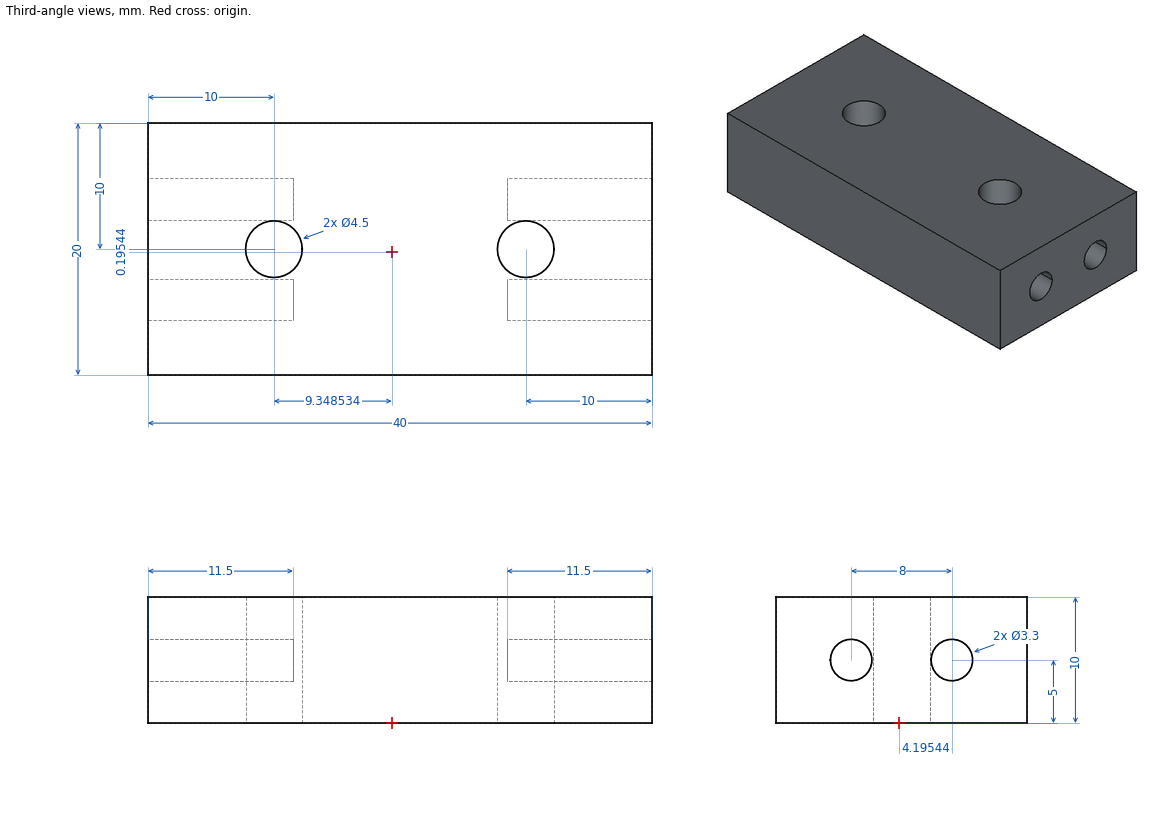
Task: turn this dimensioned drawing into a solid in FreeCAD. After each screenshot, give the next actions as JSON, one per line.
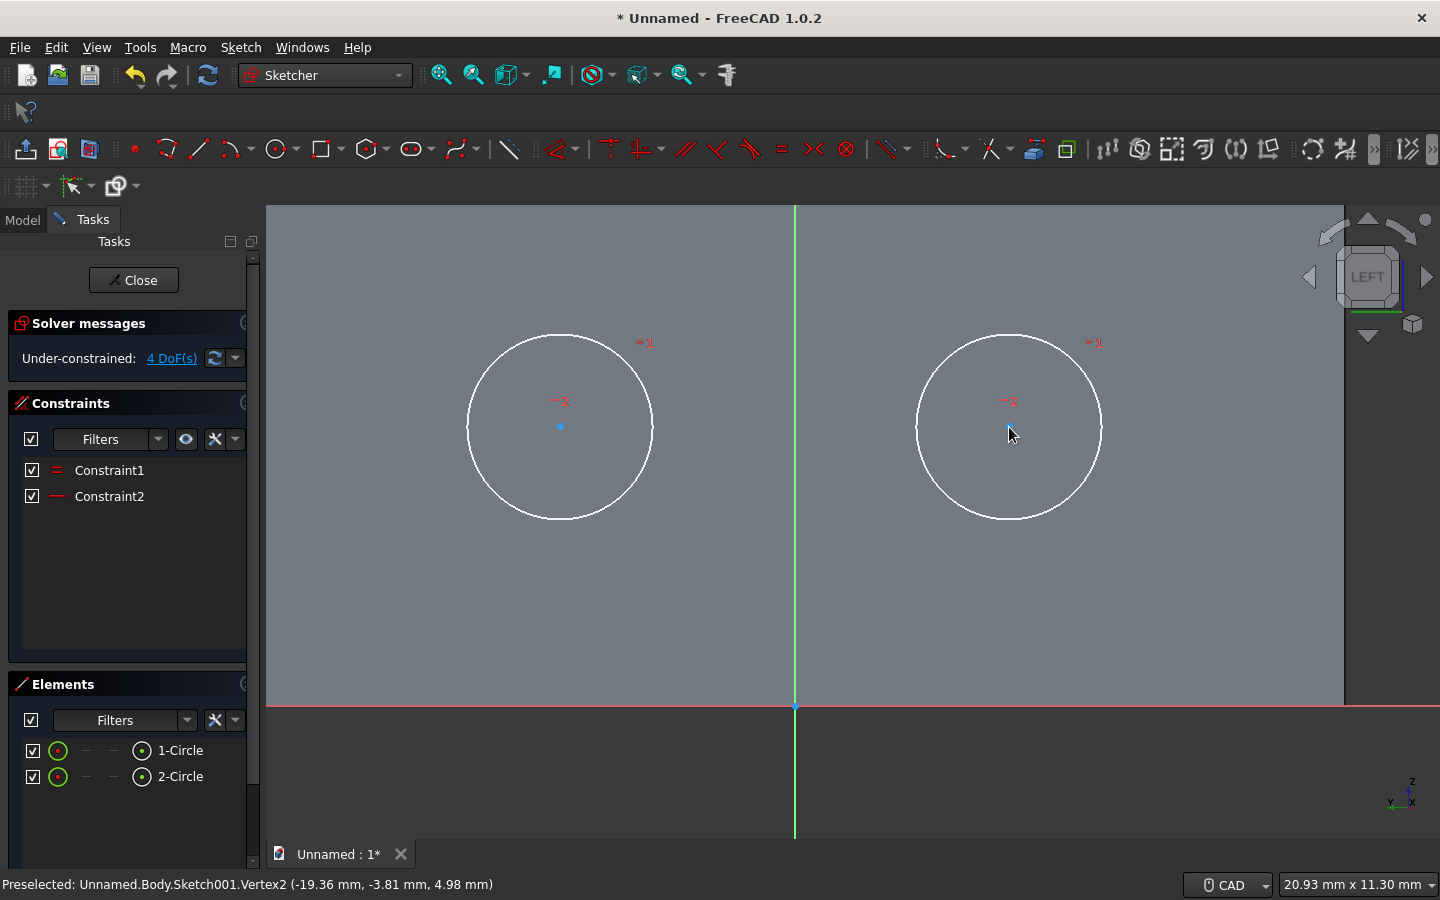
{"action": "left_click", "coordinate": [556, 150]}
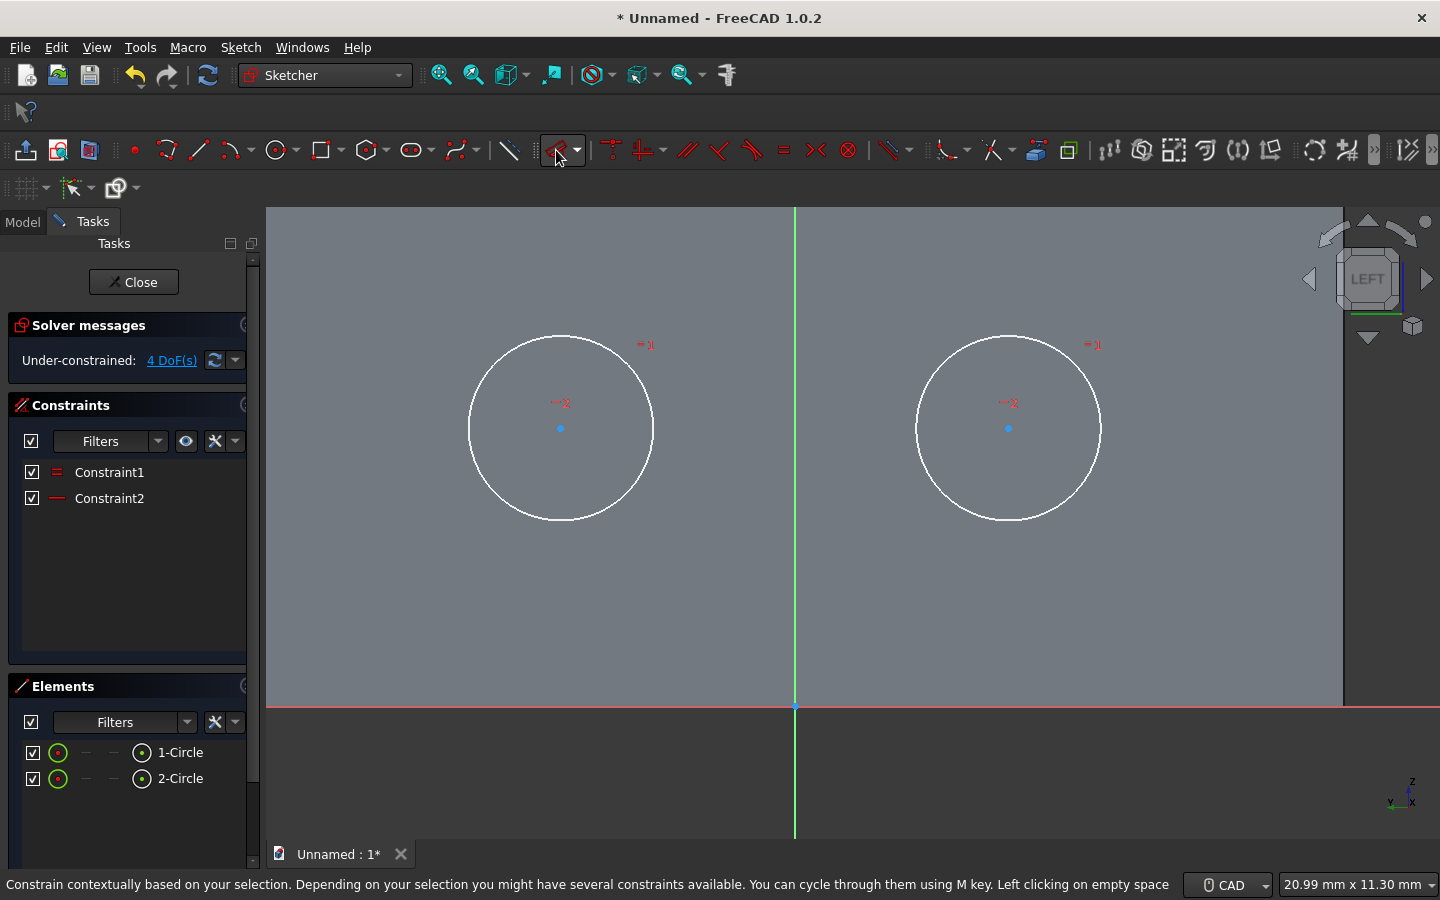
{"action": "left_click", "coordinate": [626, 363]}
{"action": "left_click", "coordinate": [649, 340]}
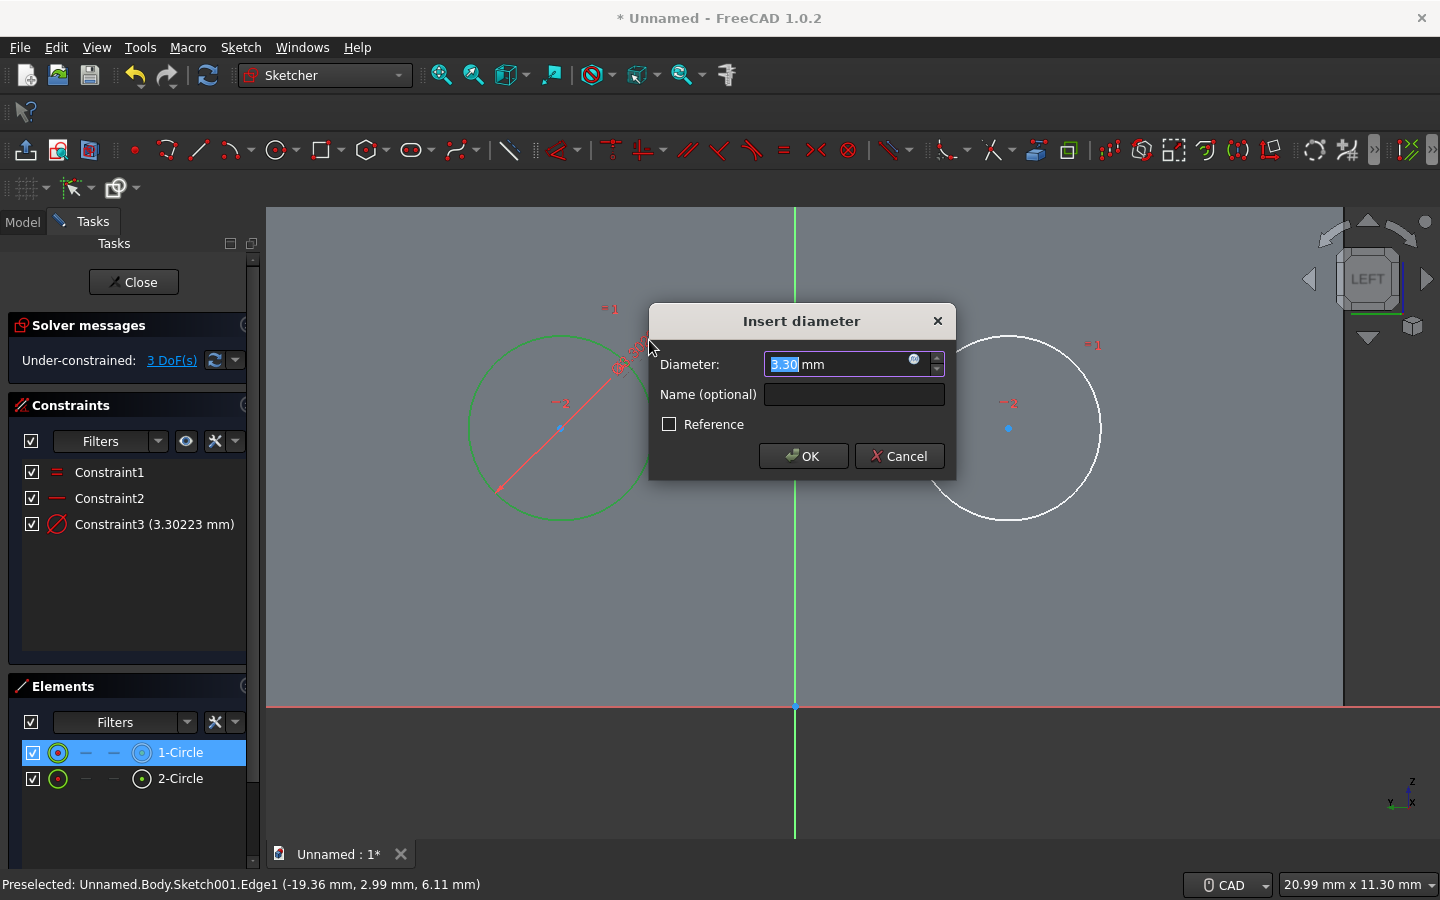
{"action": "type", "text": "3.3"}
{"action": "key", "text": "Return"}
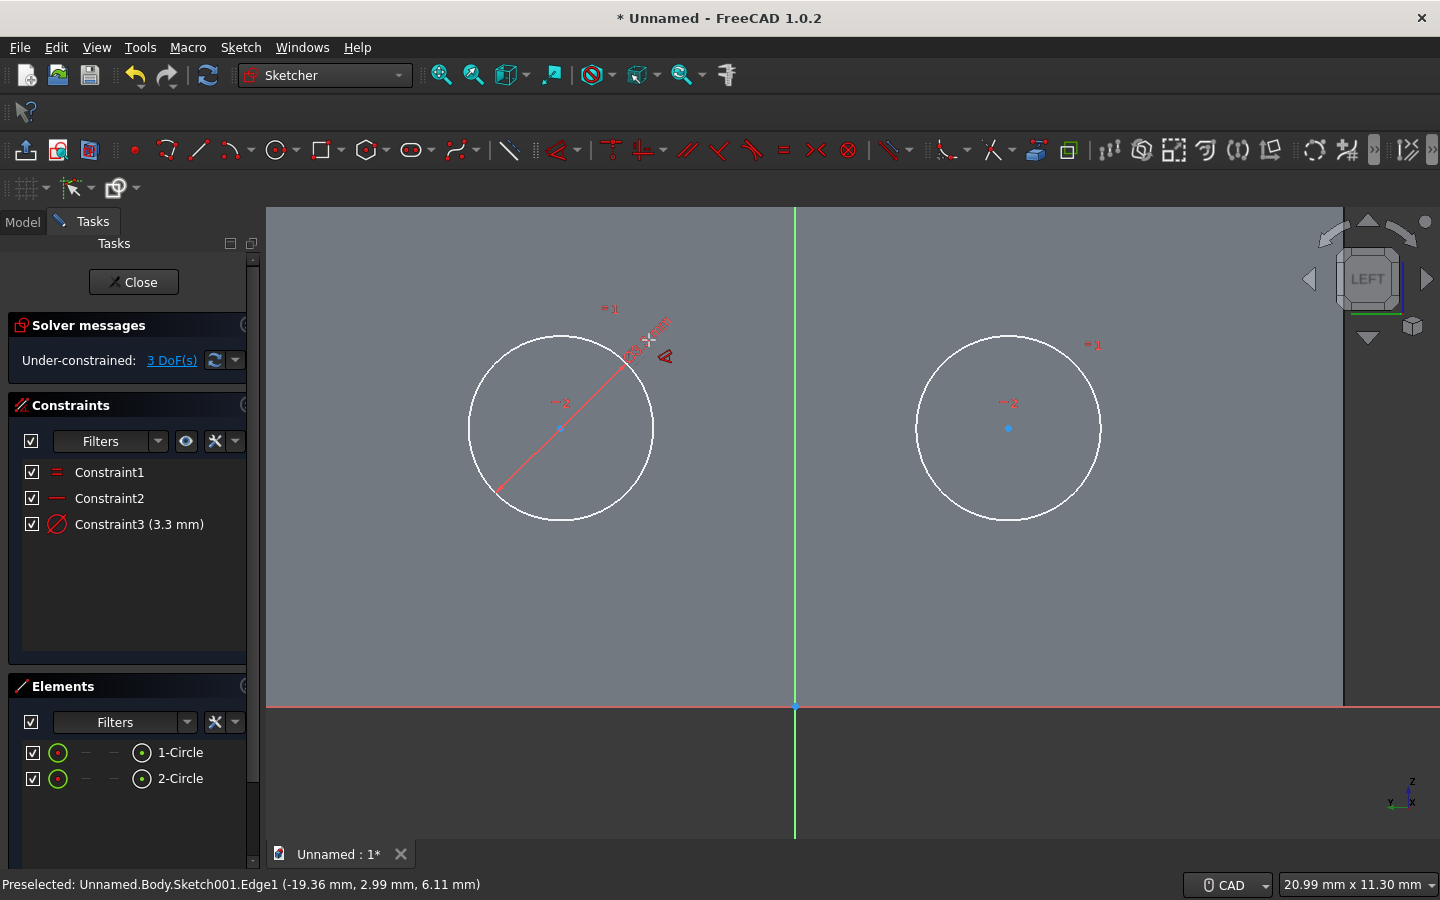
{"action": "left_click", "coordinate": [561, 428]}
{"action": "left_click", "coordinate": [527, 567]}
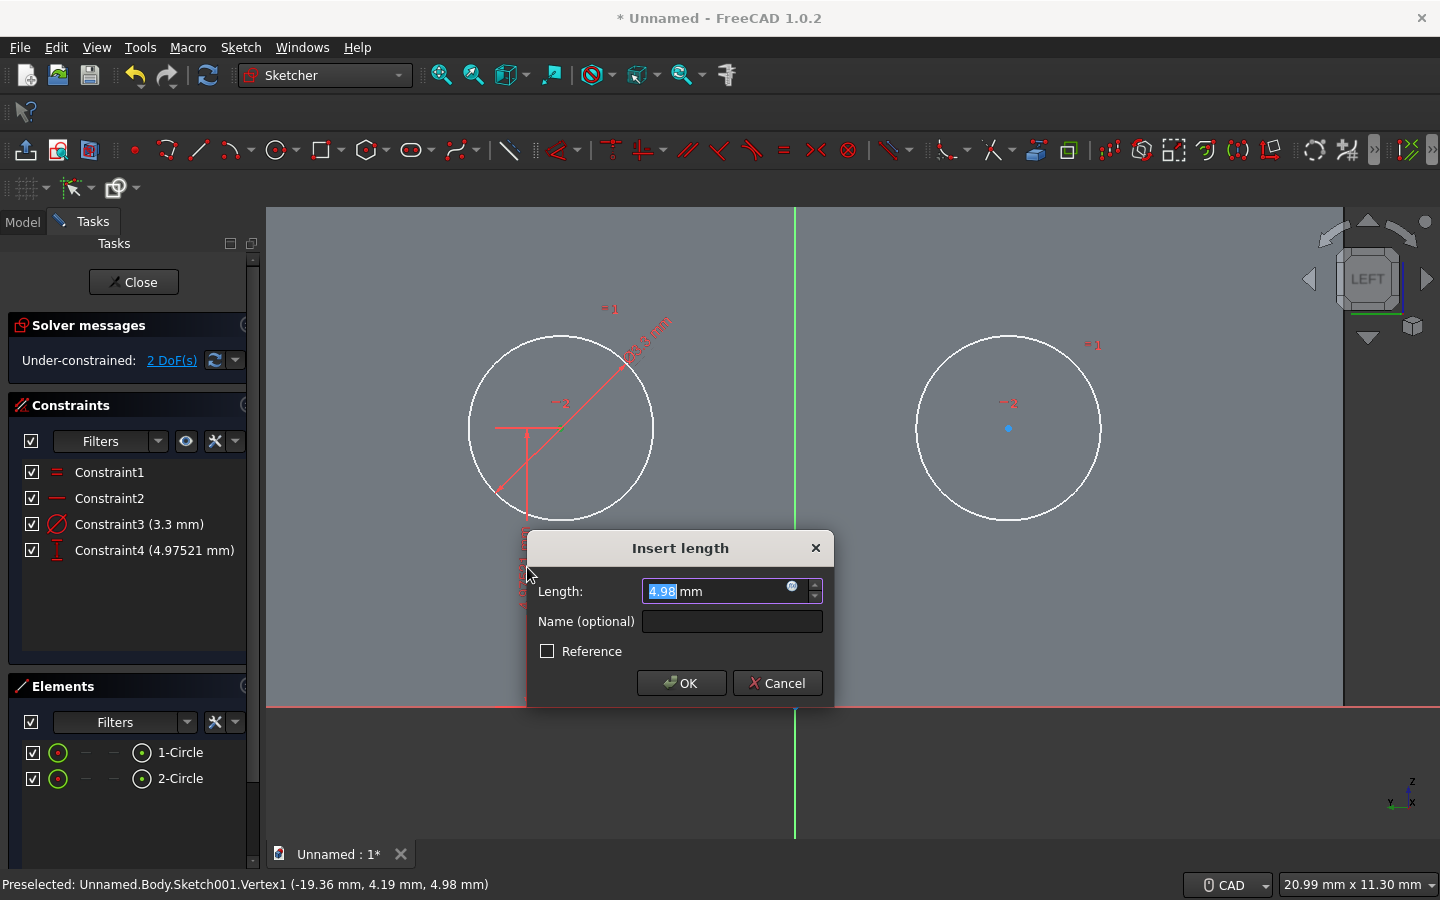
{"action": "type", "text": "5"}
{"action": "key", "text": "Return"}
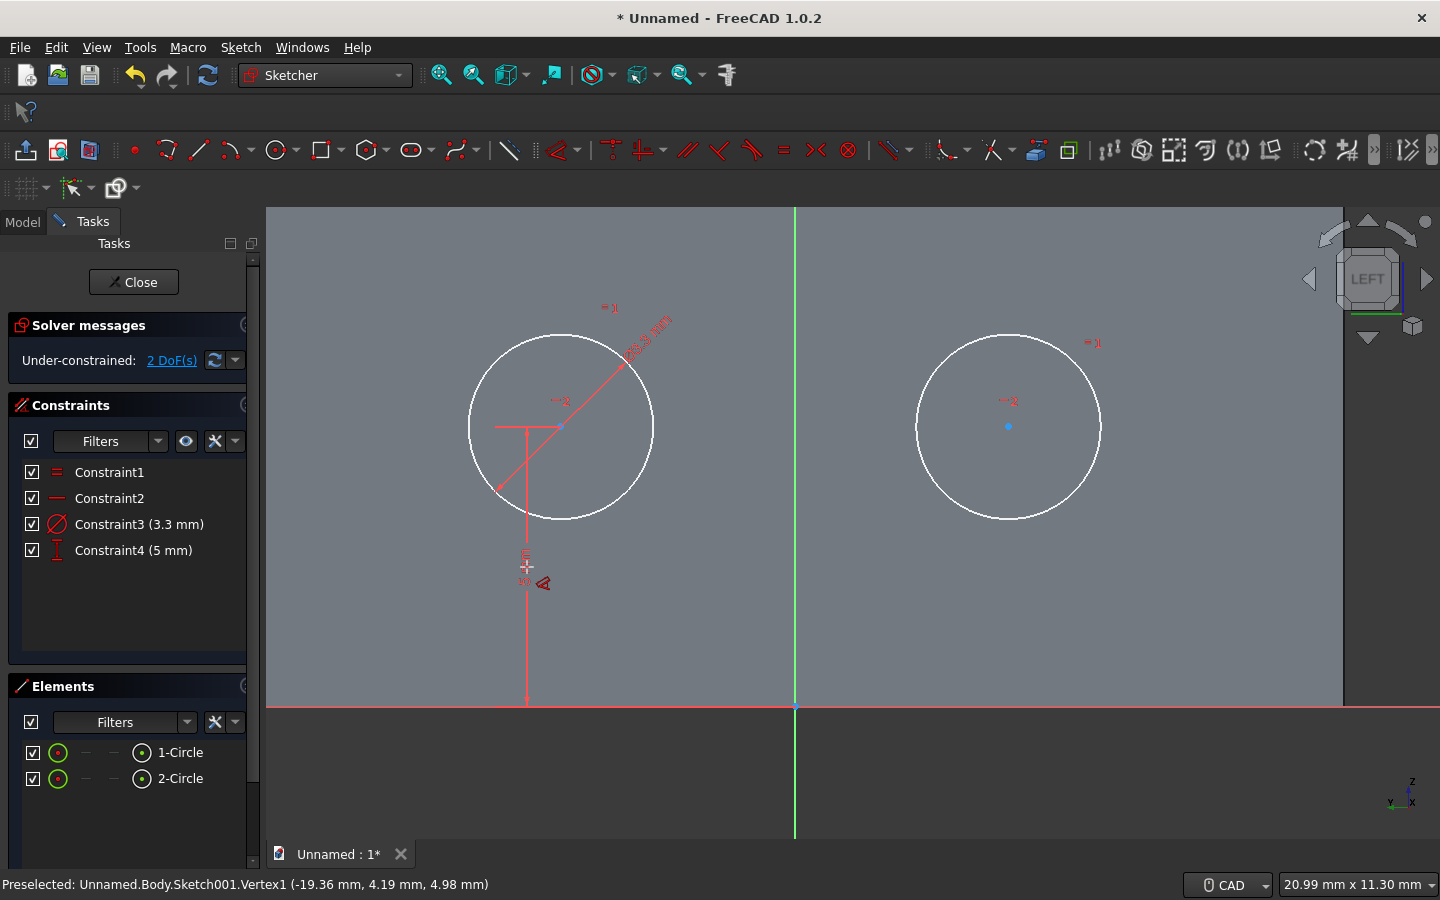
{"action": "left_click", "coordinate": [561, 427]}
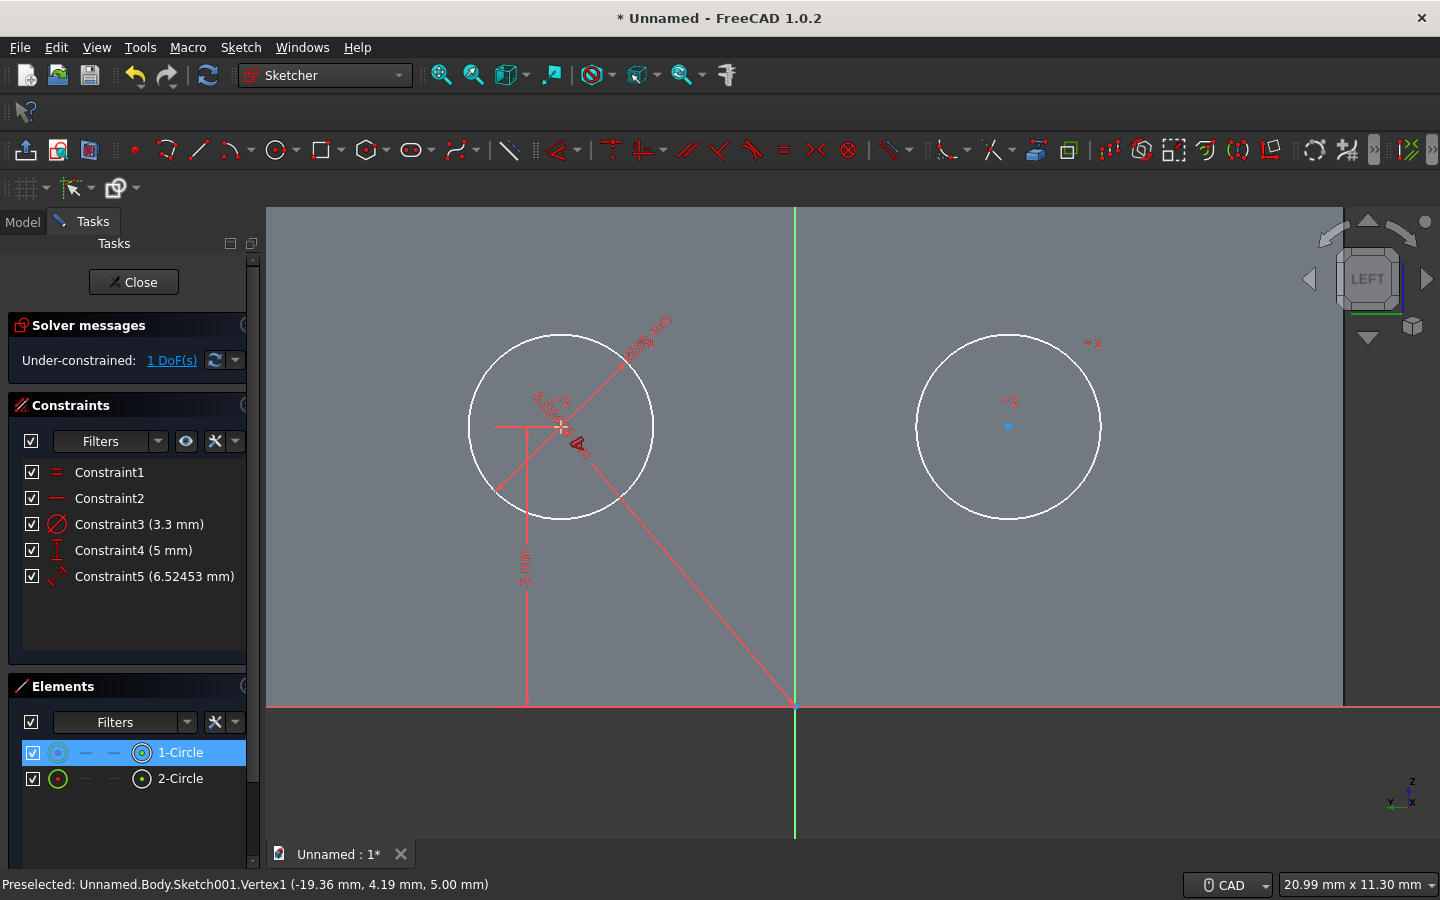
{"action": "left_click", "coordinate": [1009, 427]}
{"action": "left_click", "coordinate": [682, 393]}